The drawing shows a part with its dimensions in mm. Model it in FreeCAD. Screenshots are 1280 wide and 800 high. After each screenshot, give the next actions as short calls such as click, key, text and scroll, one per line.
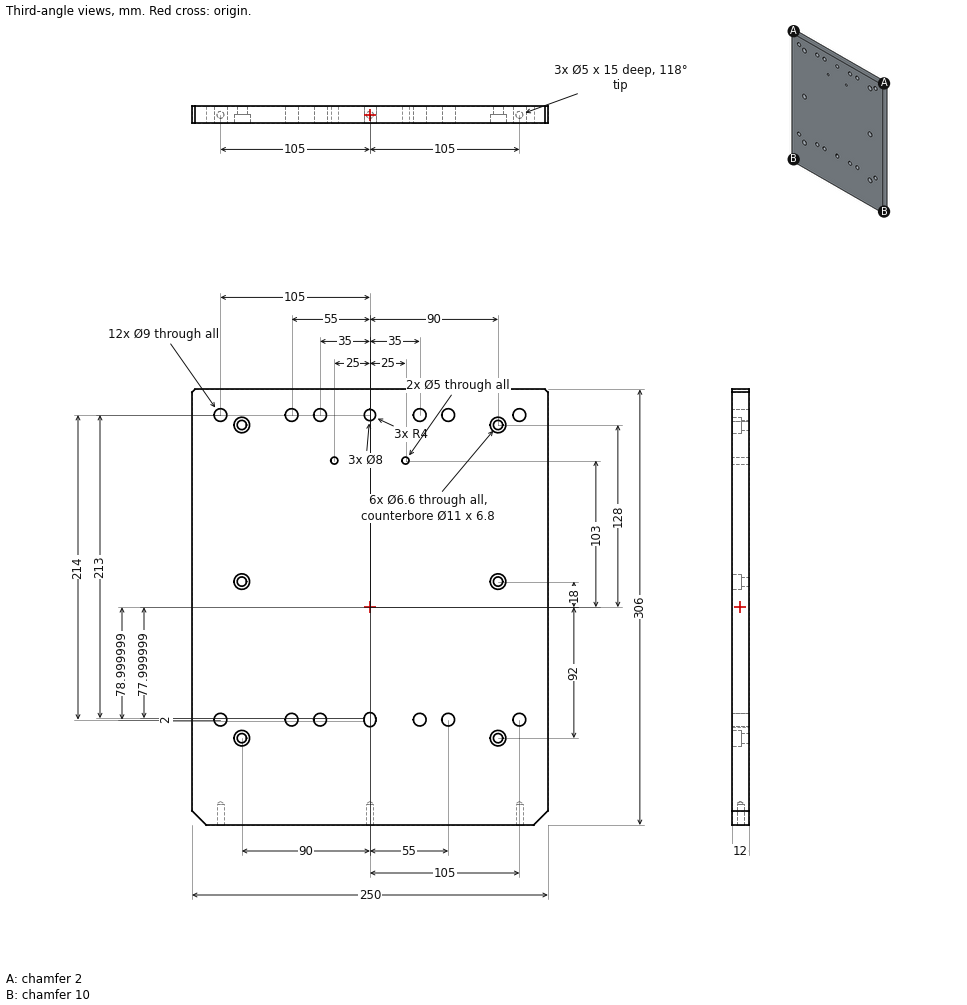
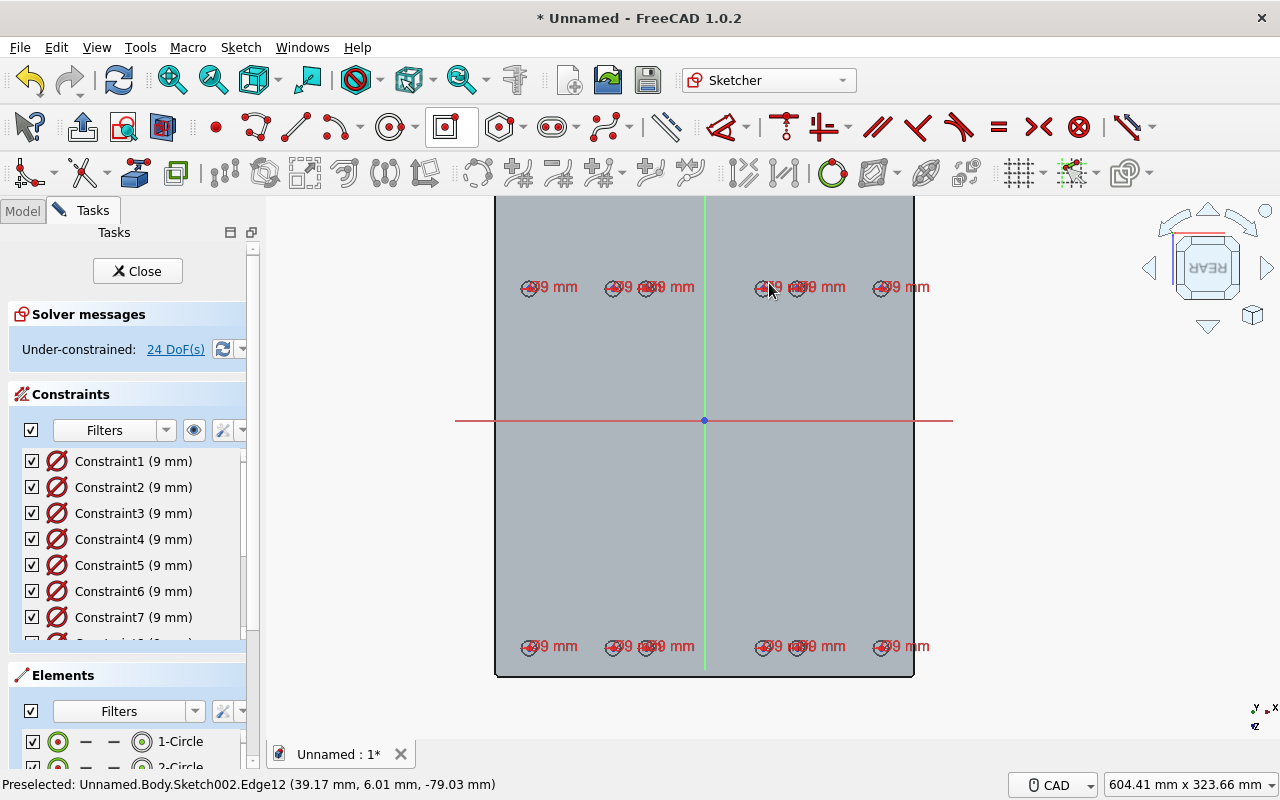
click(529, 648)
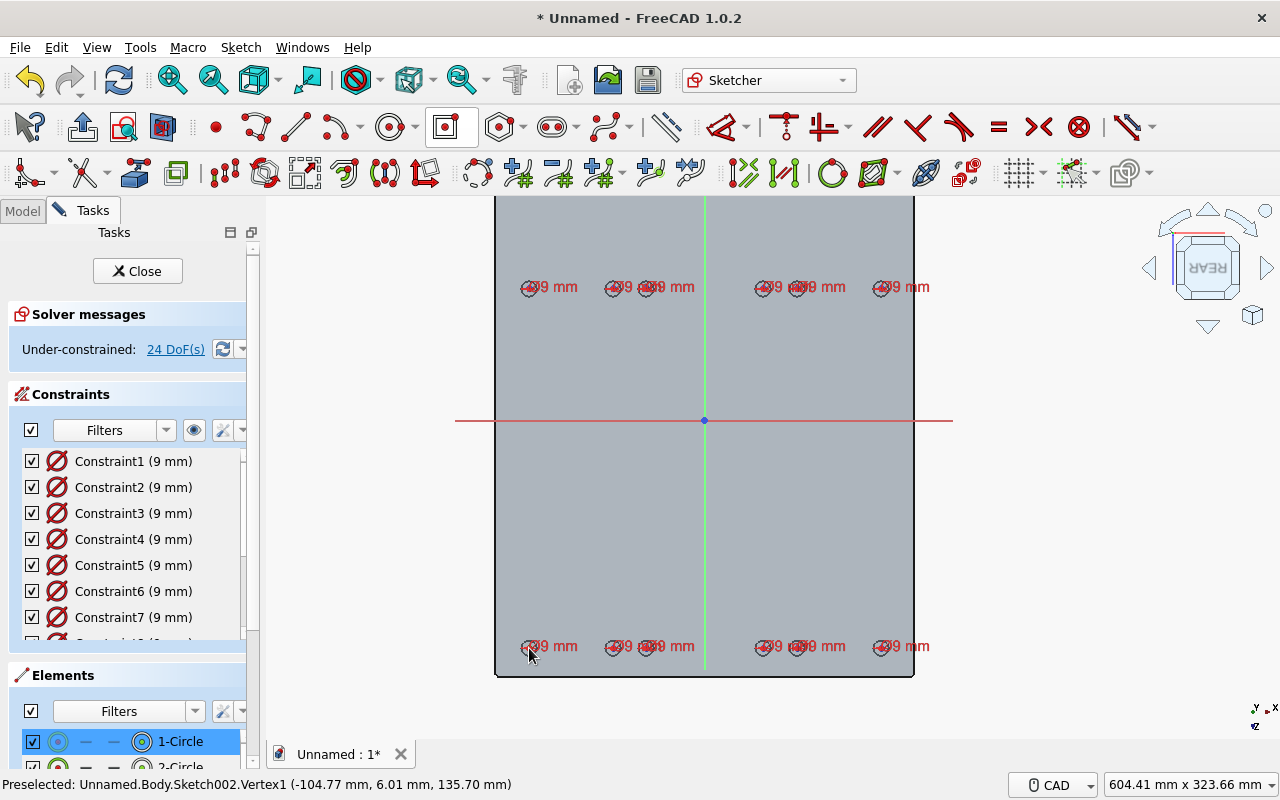
click(613, 648)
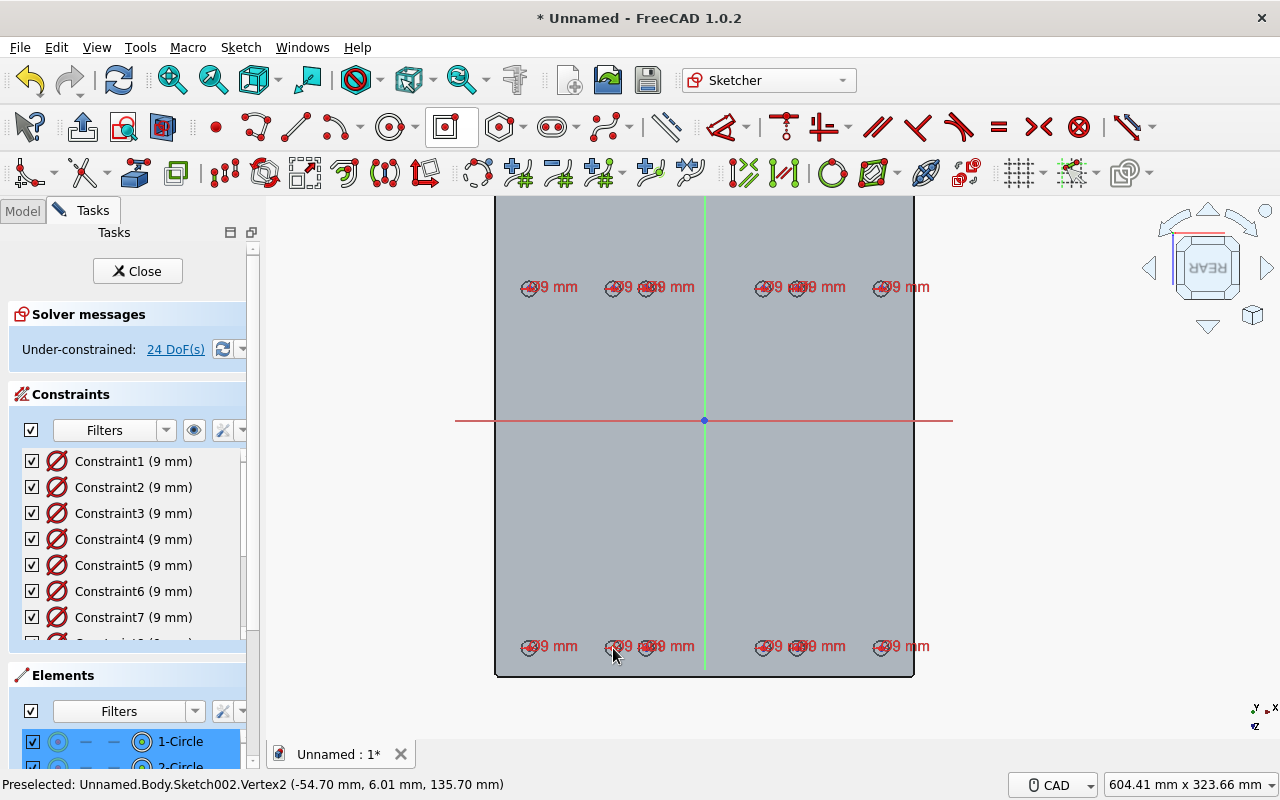
click(850, 128)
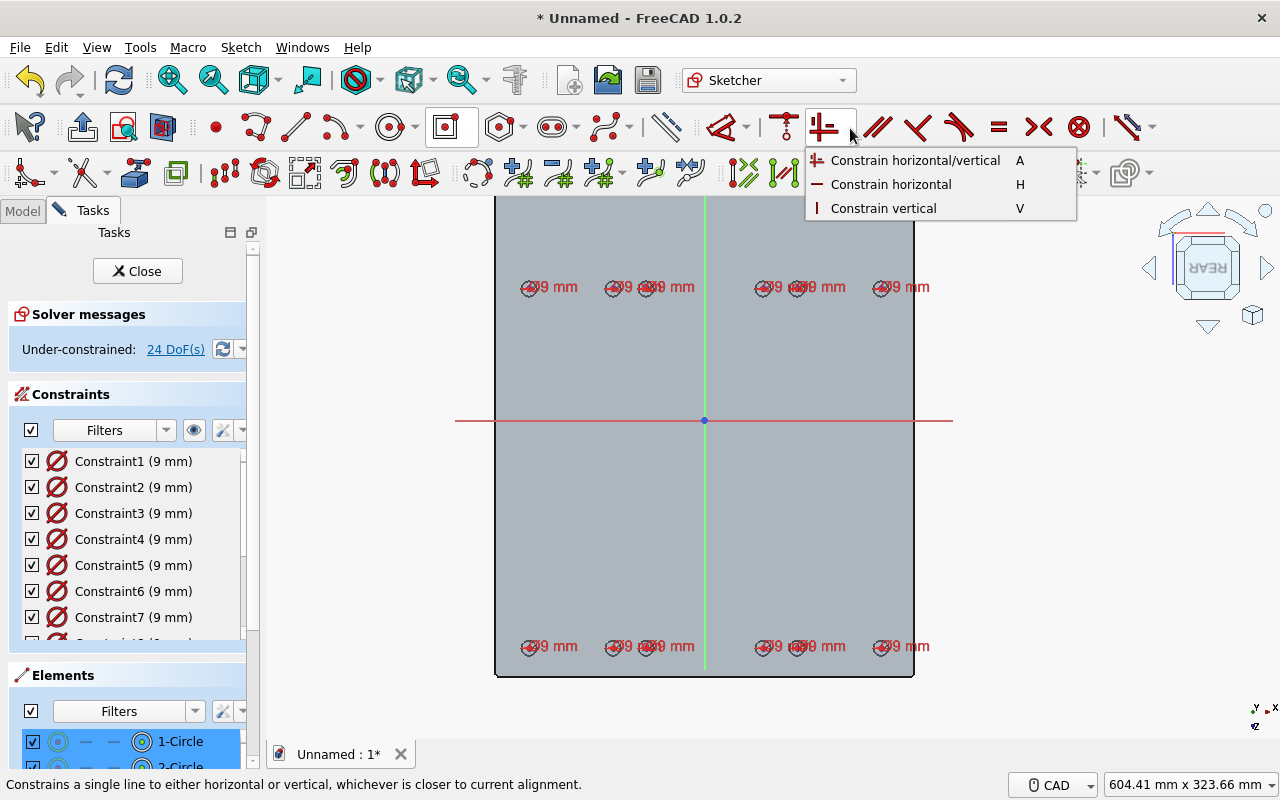
click(941, 184)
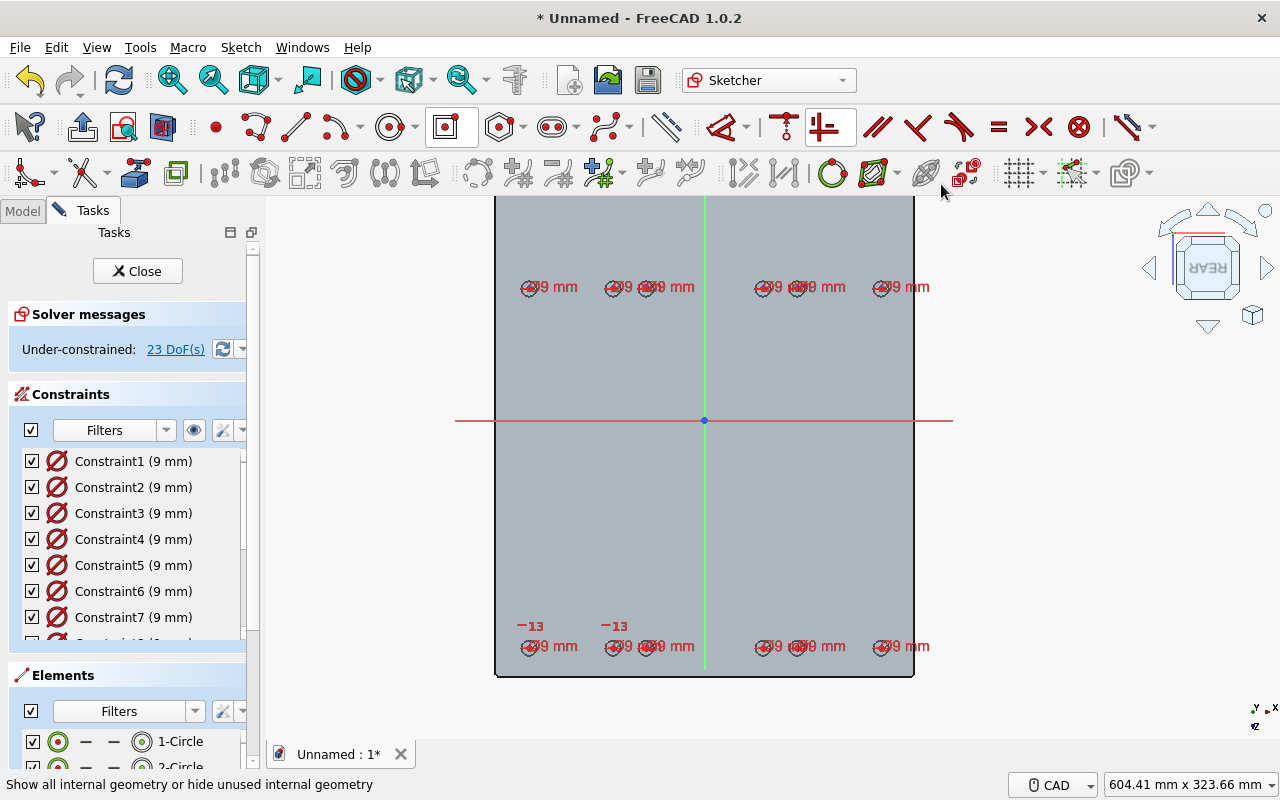
click(529, 648)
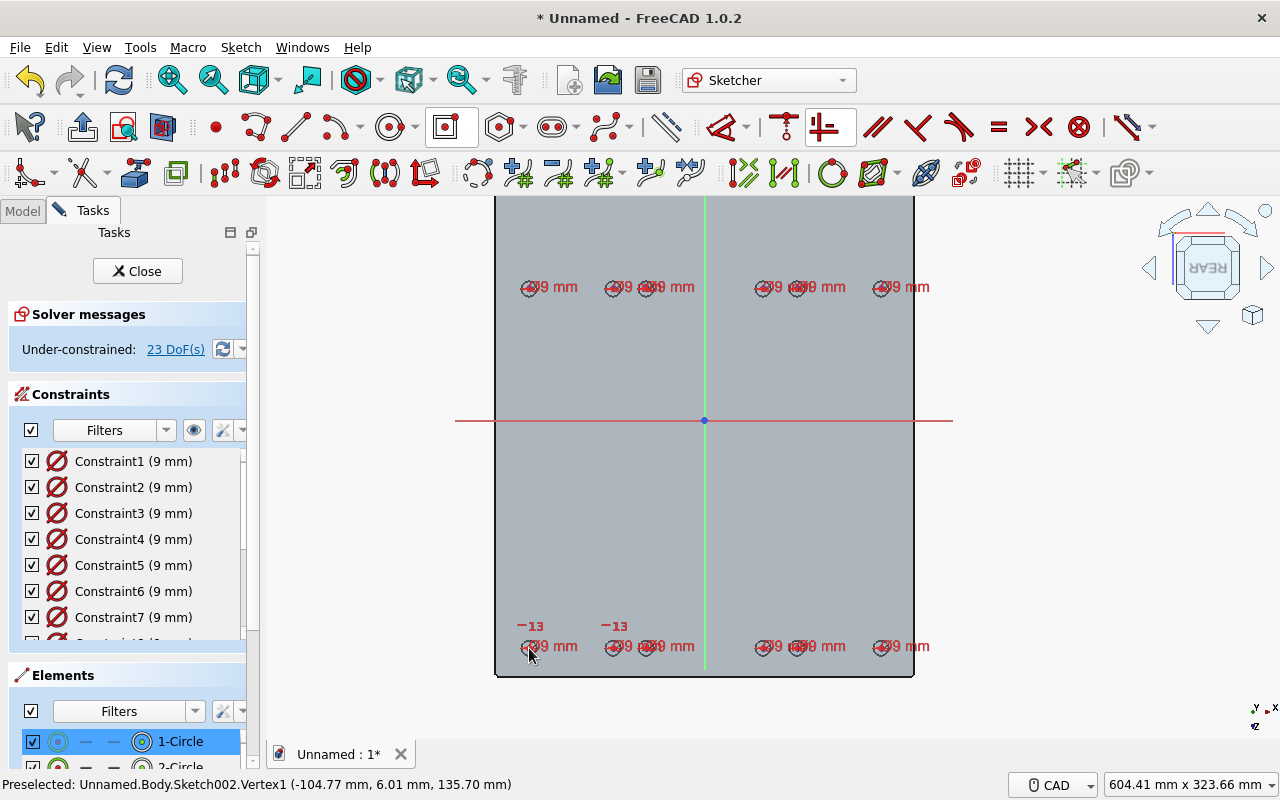
click(529, 289)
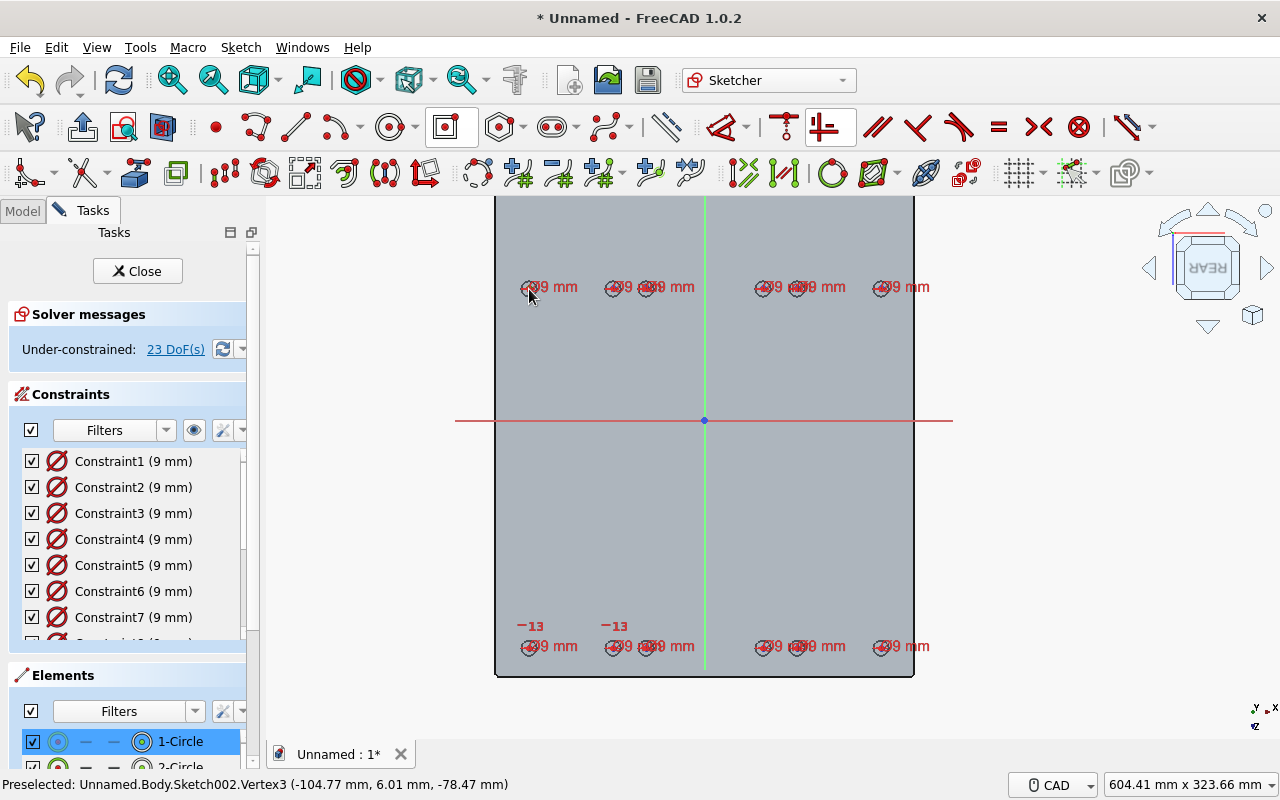
click(850, 128)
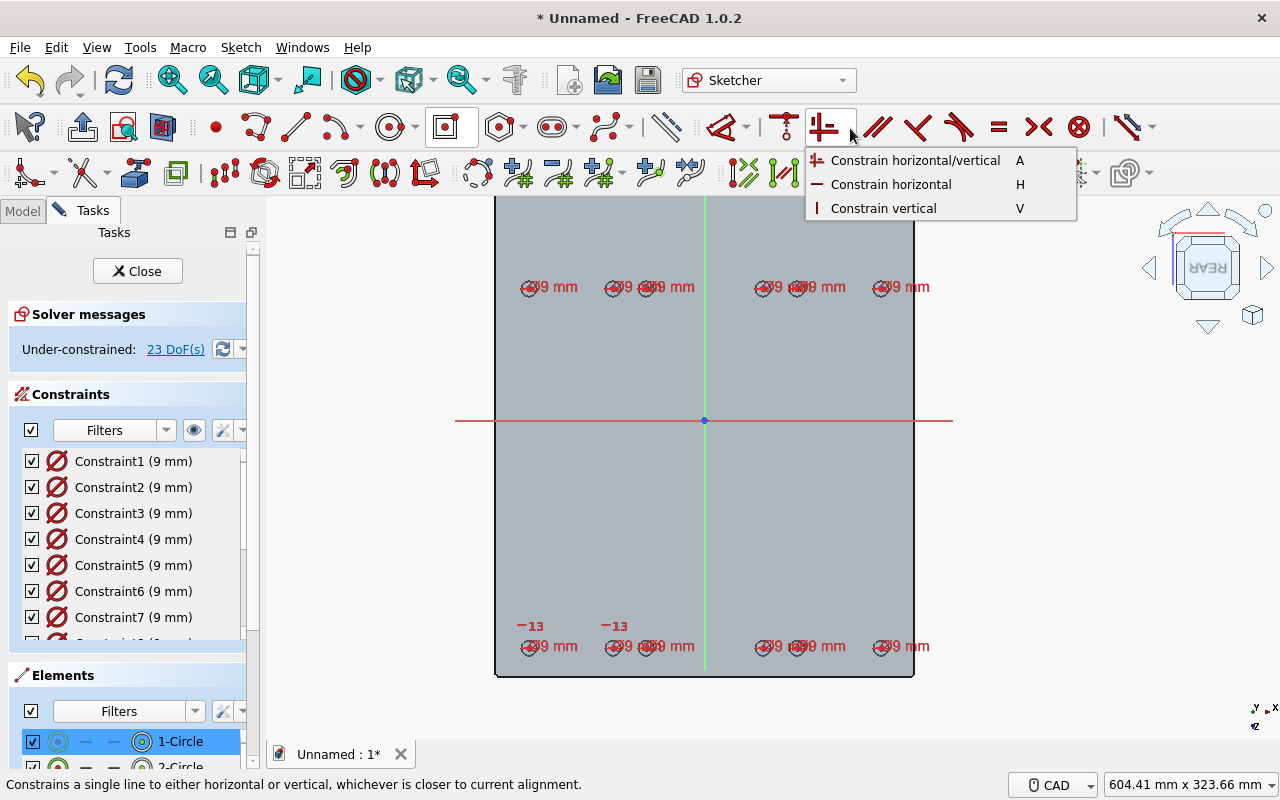
click(941, 208)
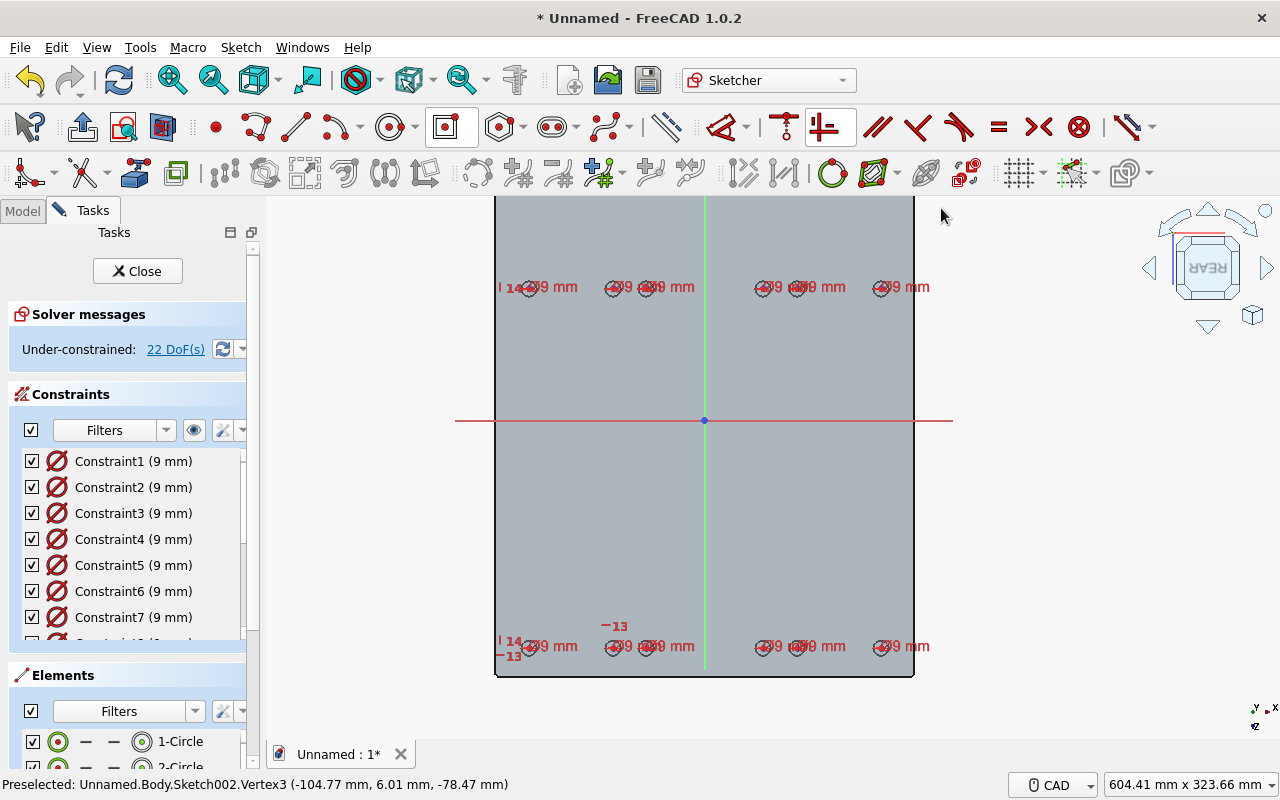
click(613, 648)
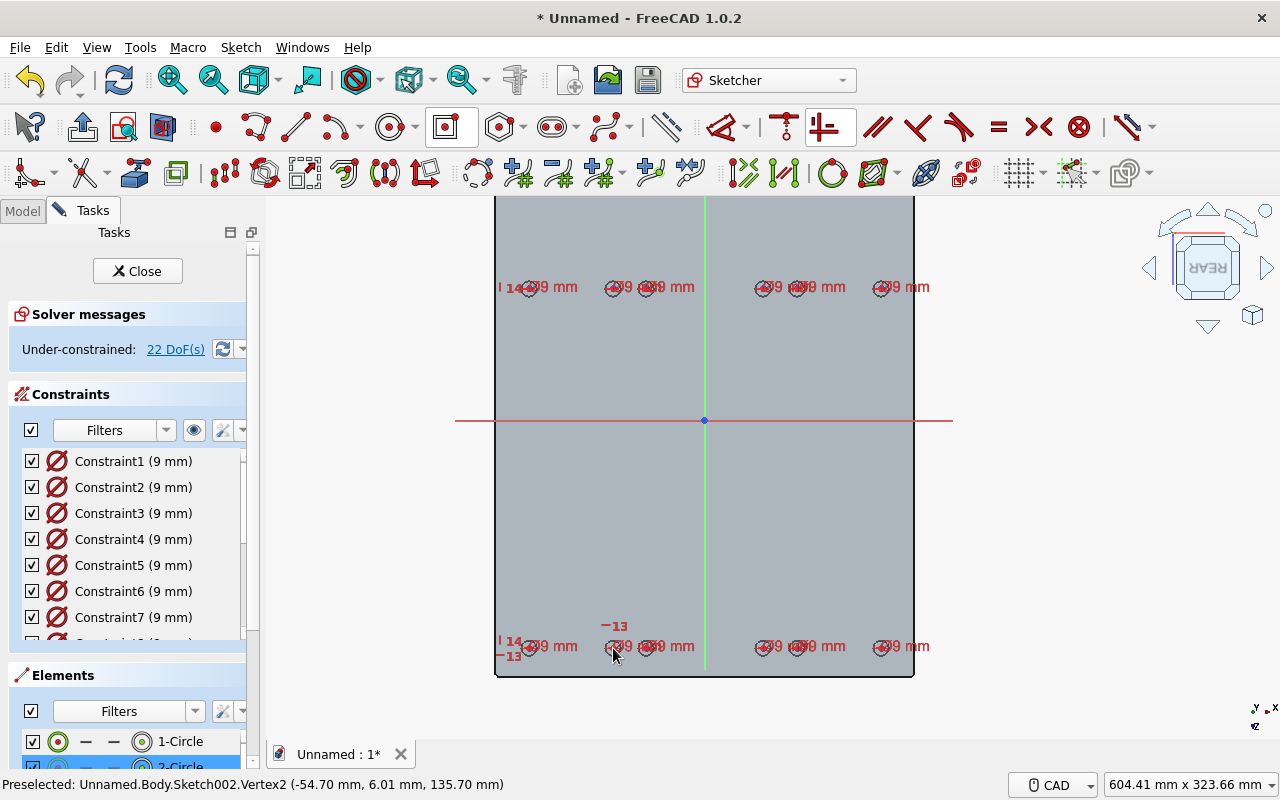
click(613, 289)